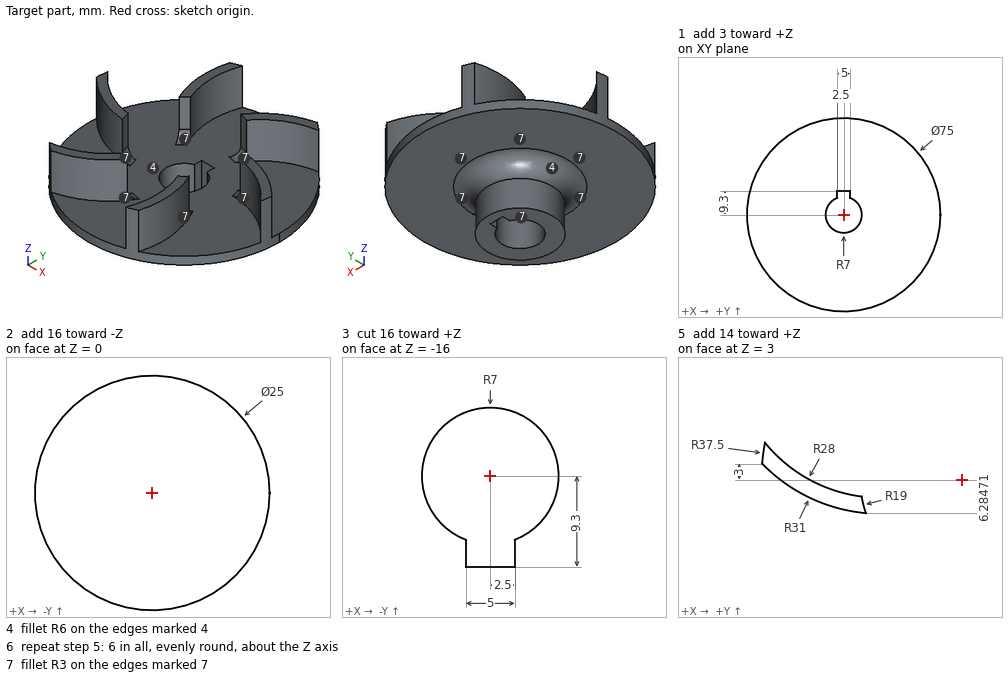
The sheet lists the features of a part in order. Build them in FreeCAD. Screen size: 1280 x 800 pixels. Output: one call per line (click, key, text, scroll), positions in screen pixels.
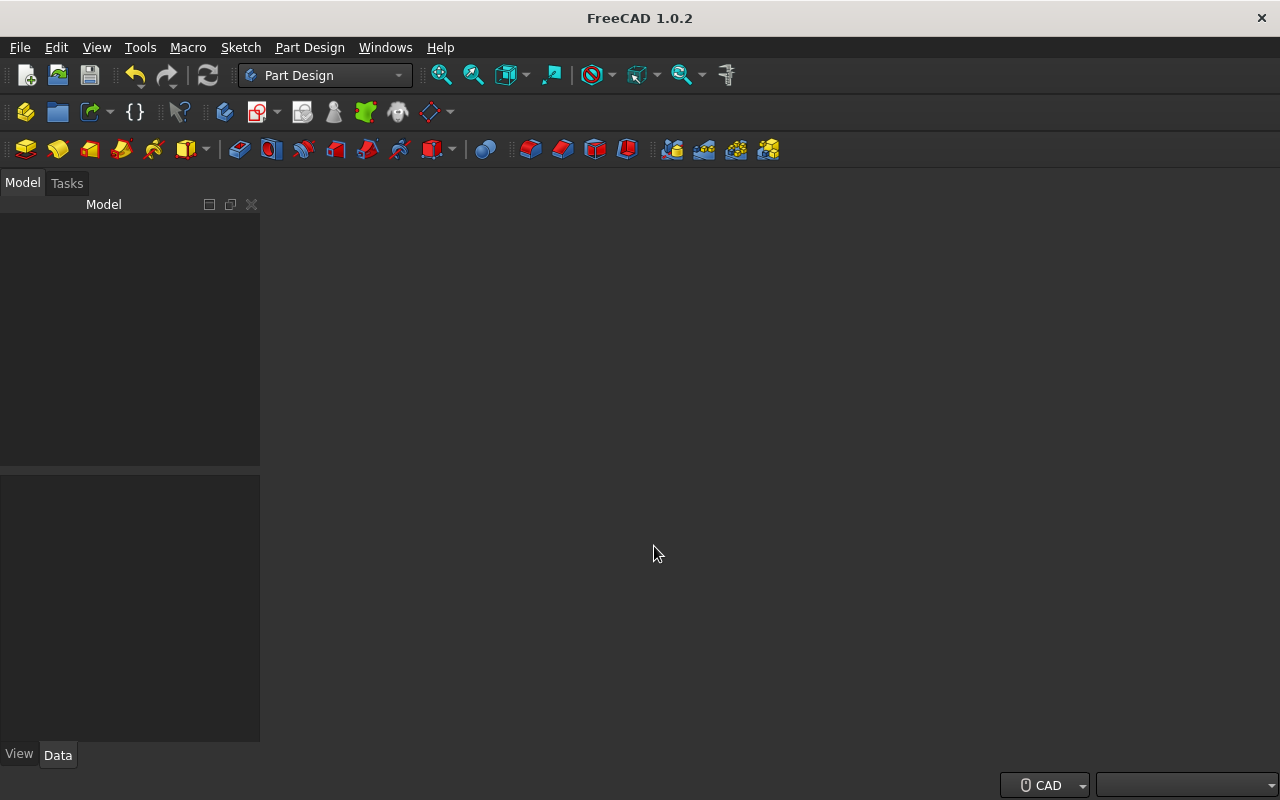
key(ctrl+n)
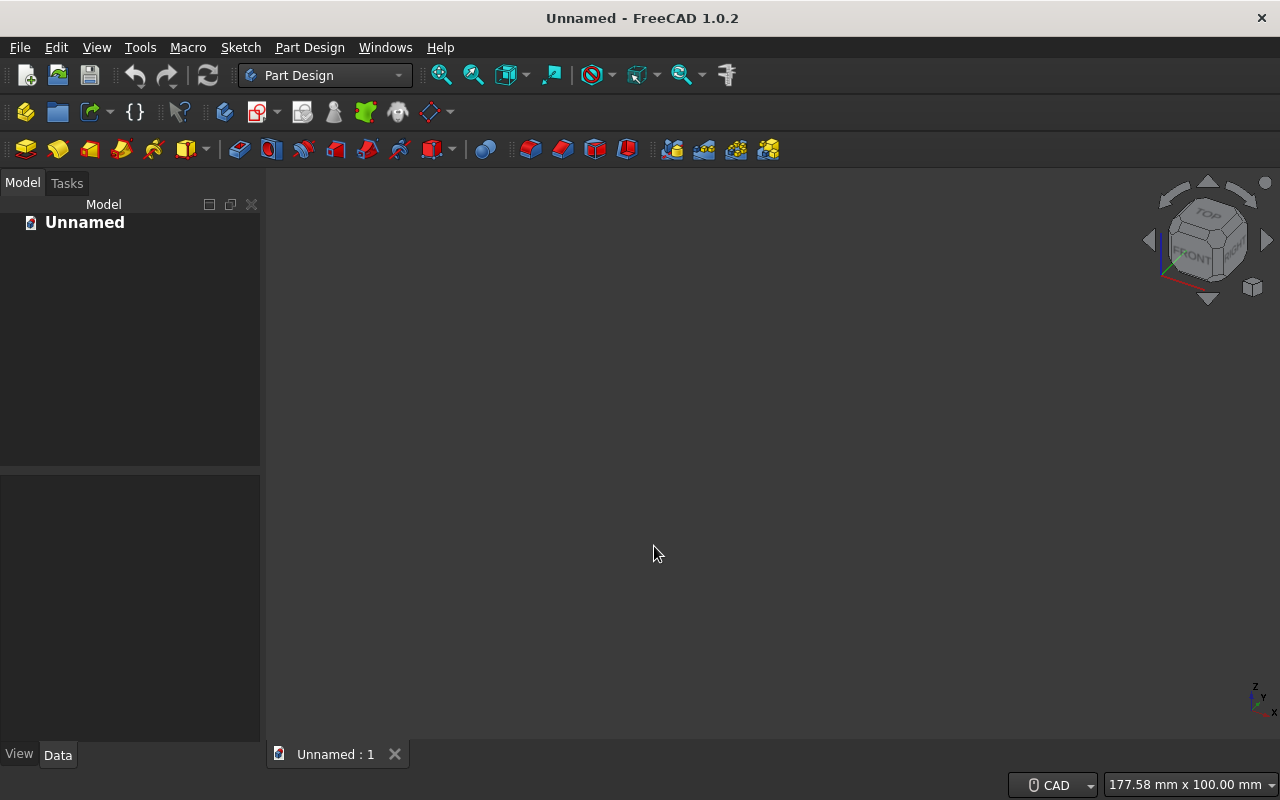
click(258, 112)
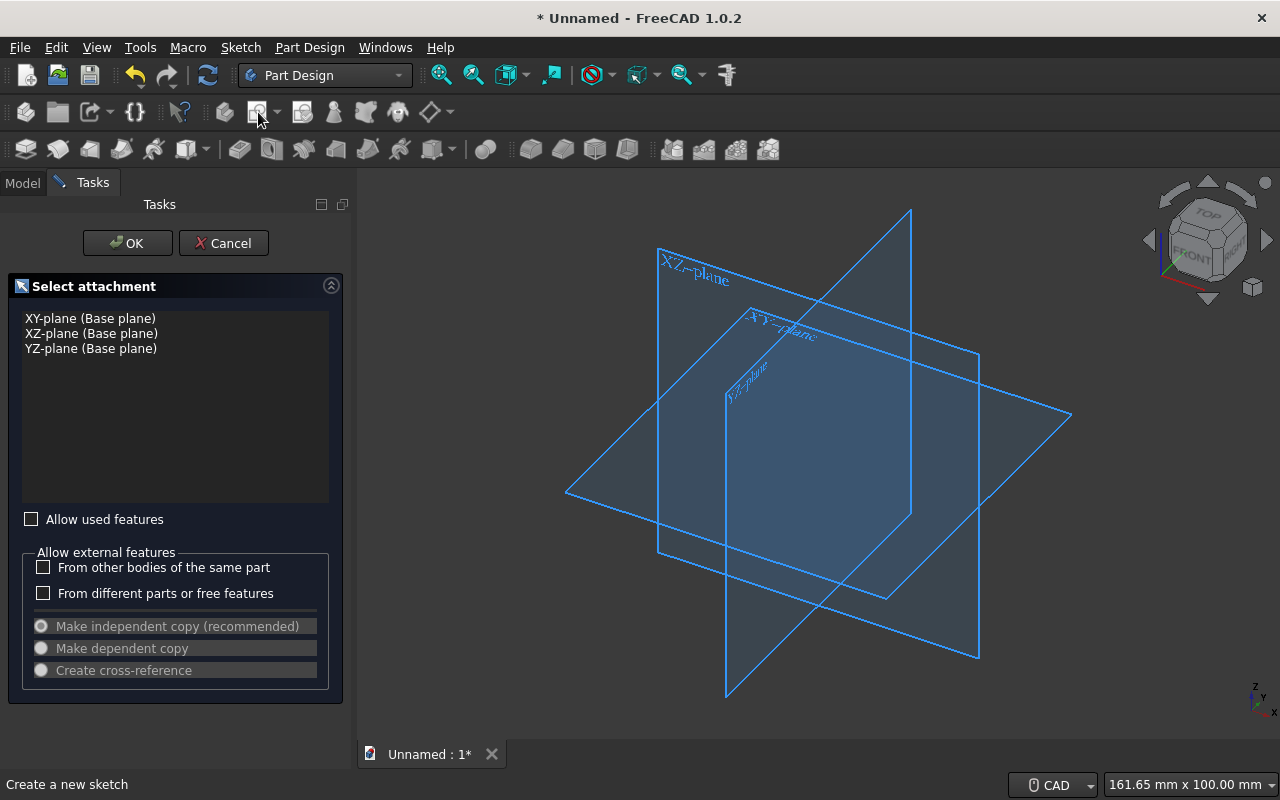
click(82, 318)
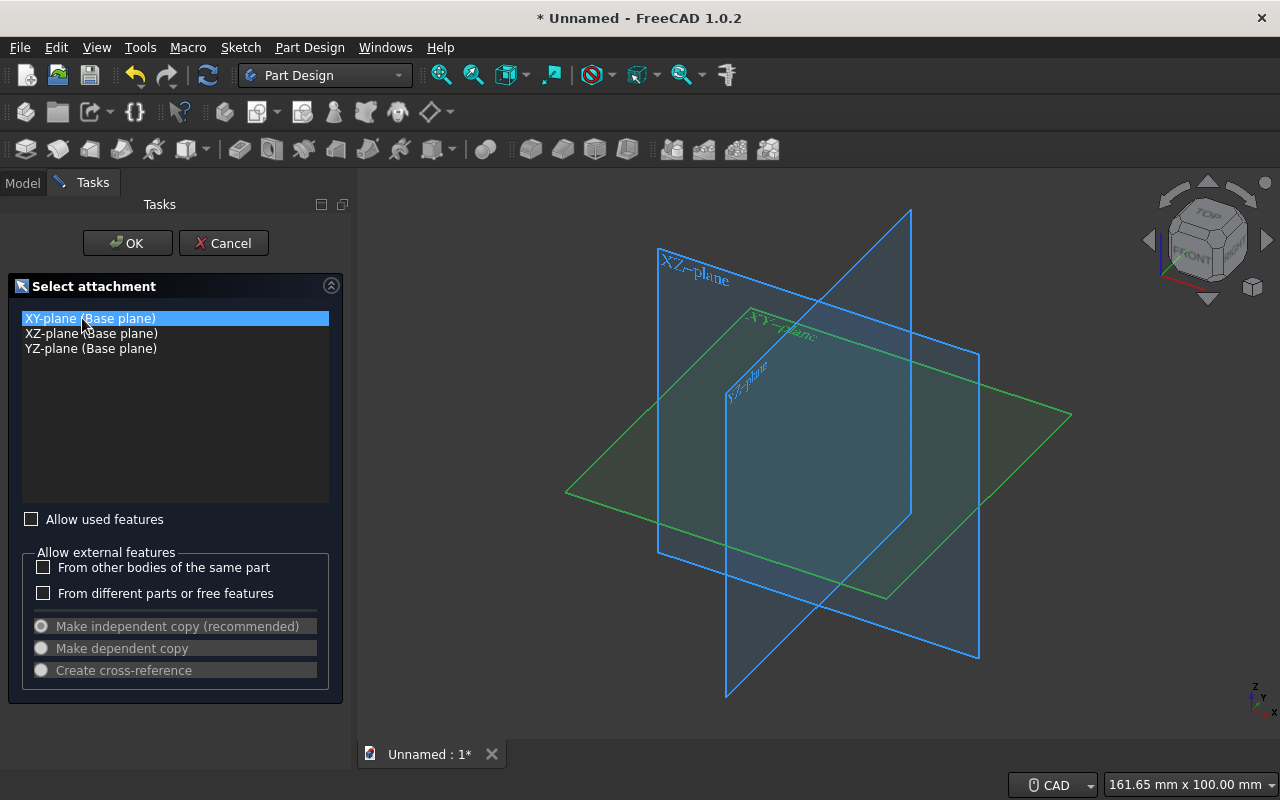
click(128, 243)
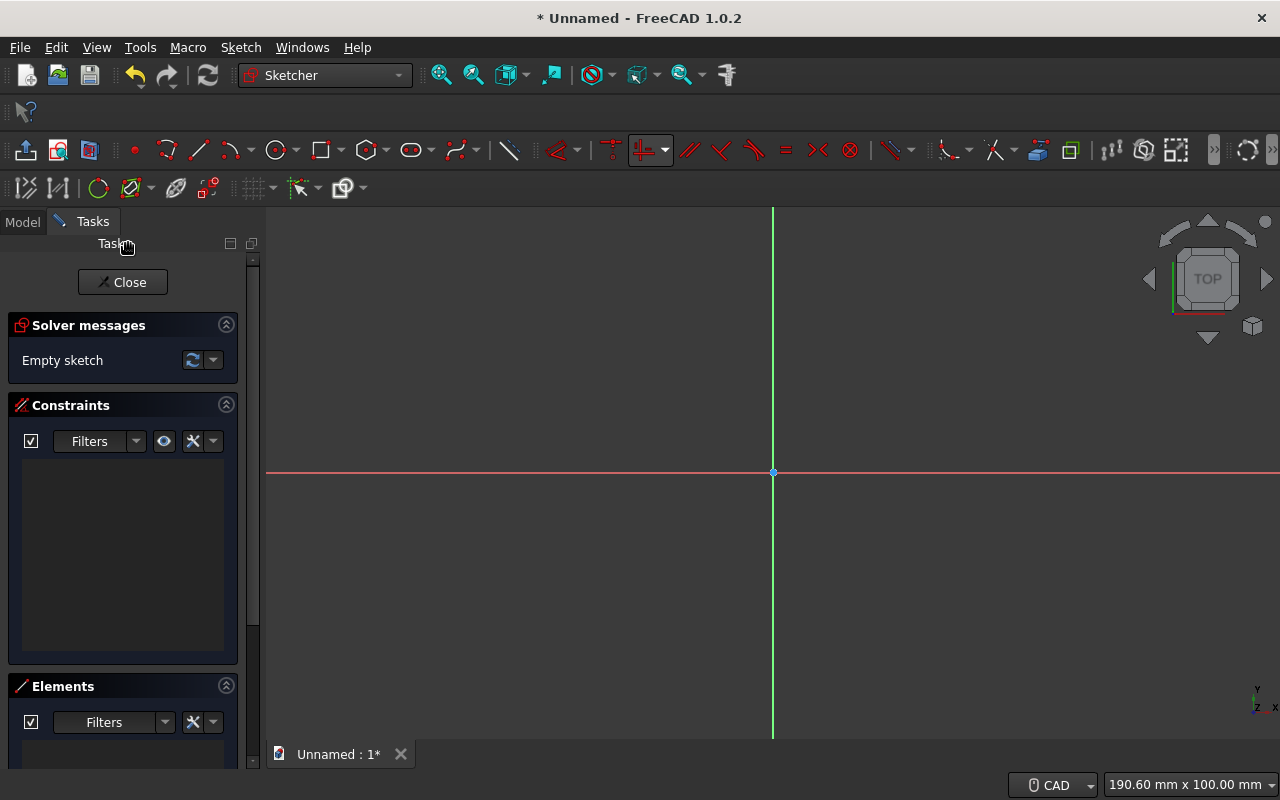
key(g)
key(m)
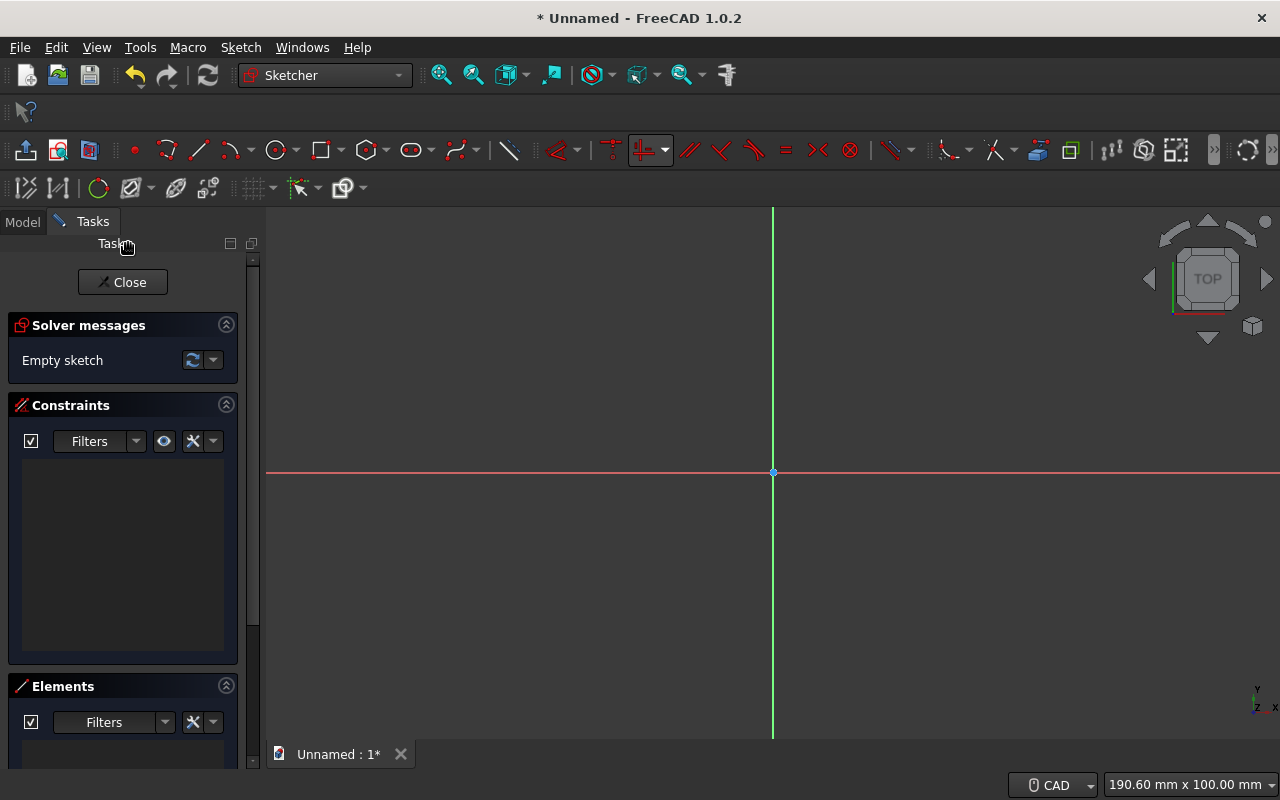
click(760, 438)
click(760, 424)
click(786, 424)
click(786, 438)
right_click(786, 438)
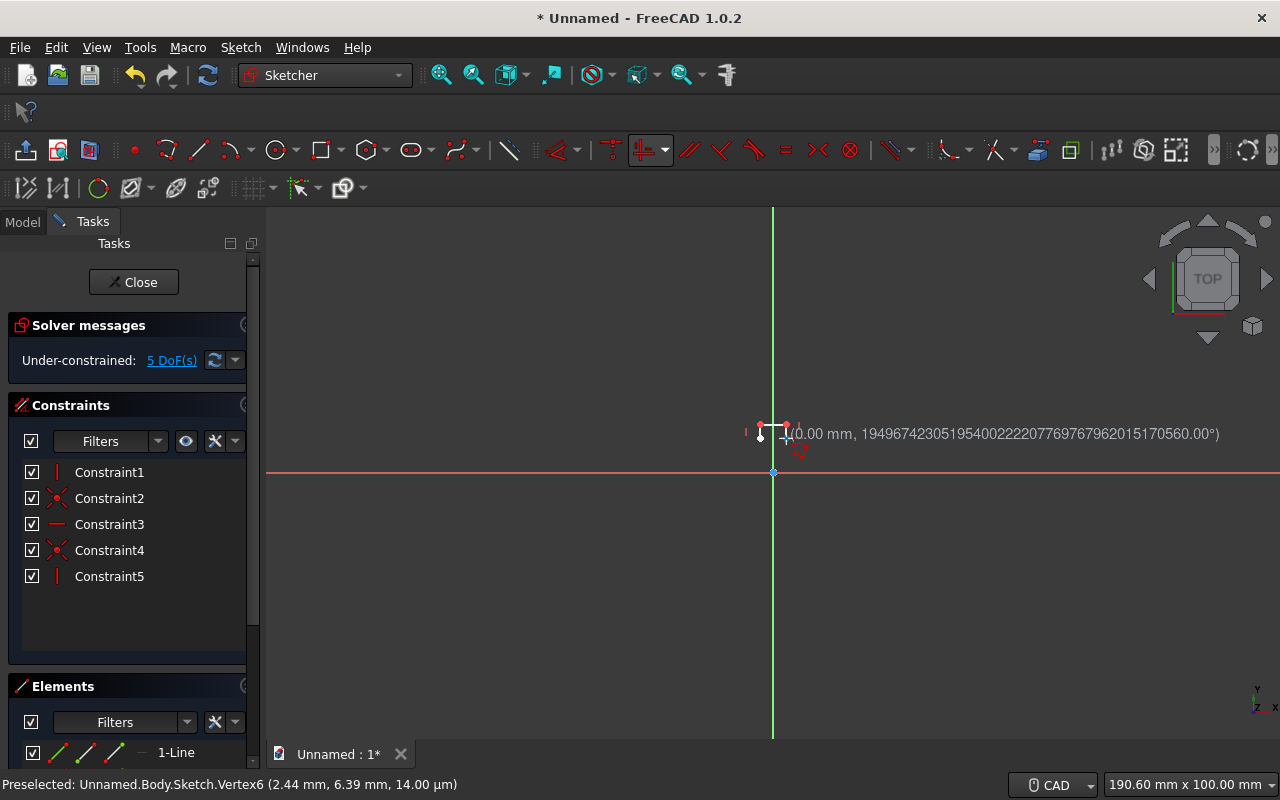
key(g)
key(3)
key(a)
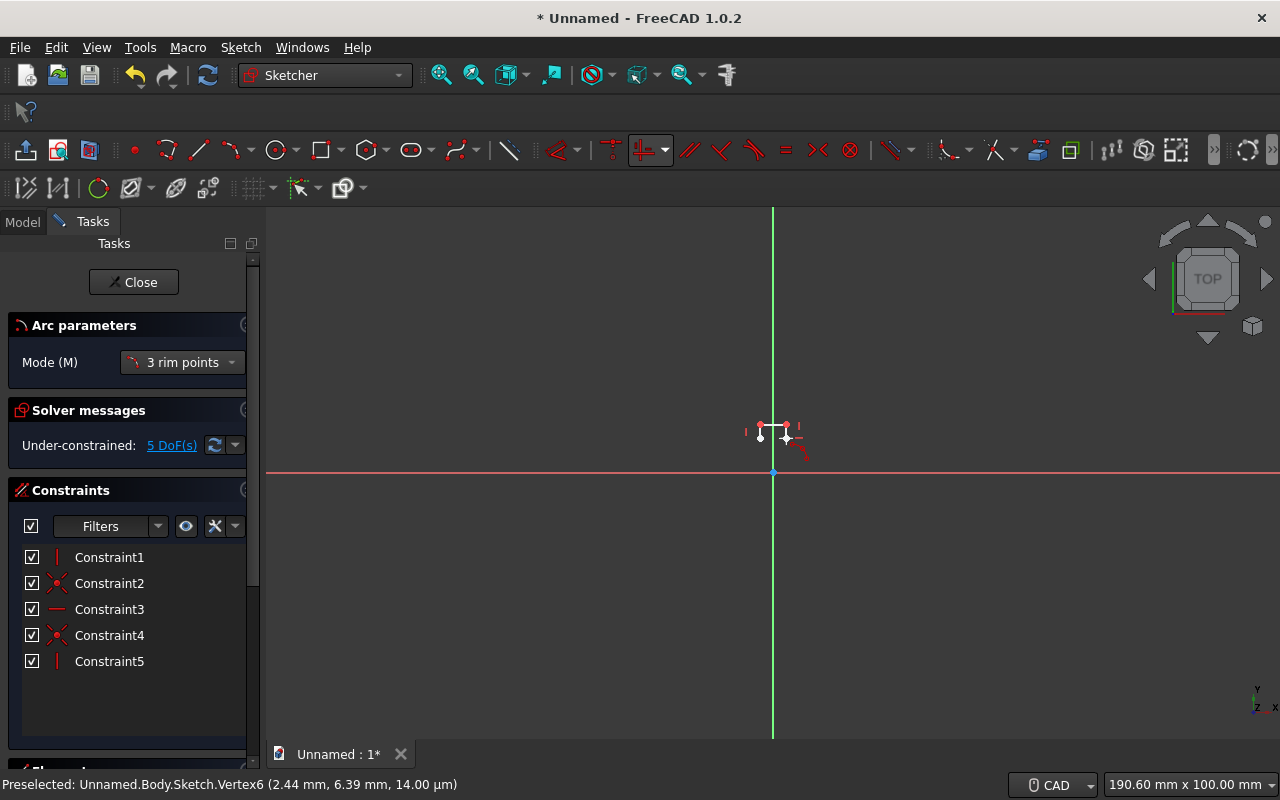
scroll(786, 438, up, 4)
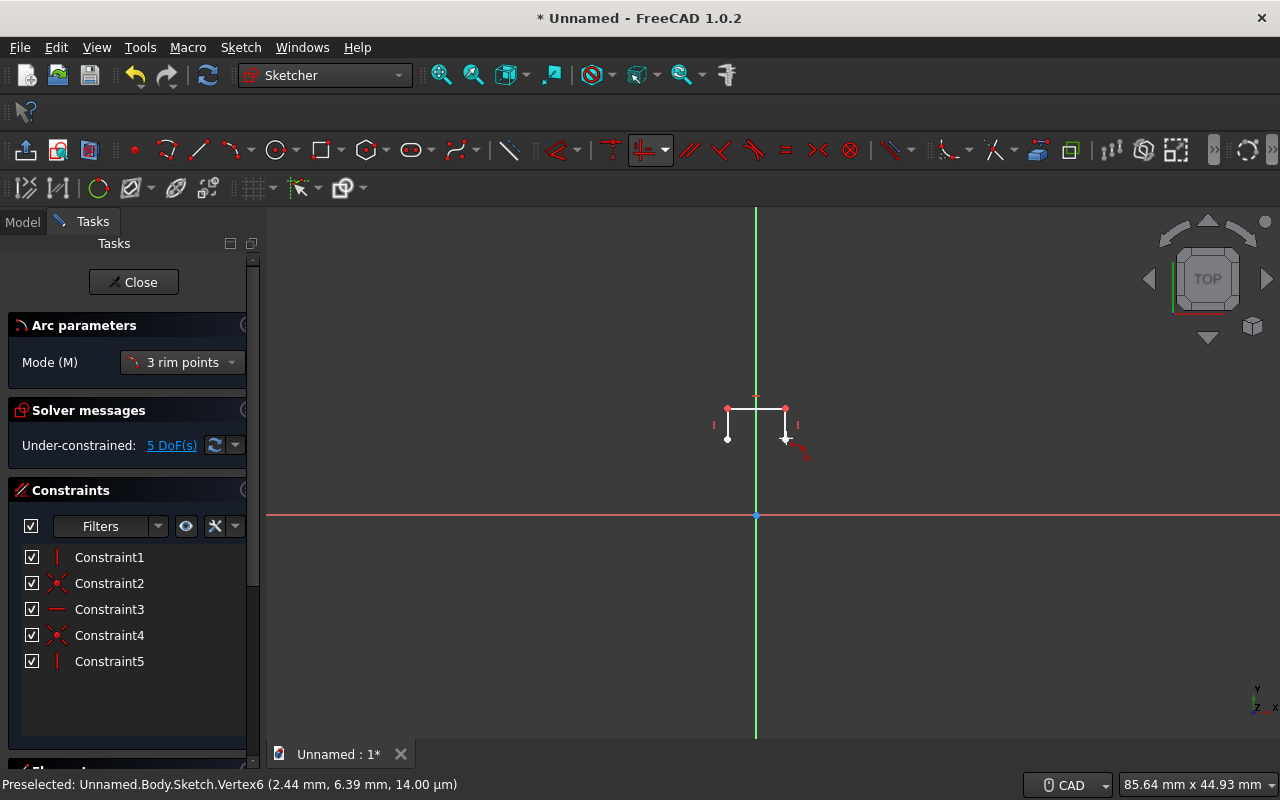
click(785, 440)
click(728, 440)
click(713, 586)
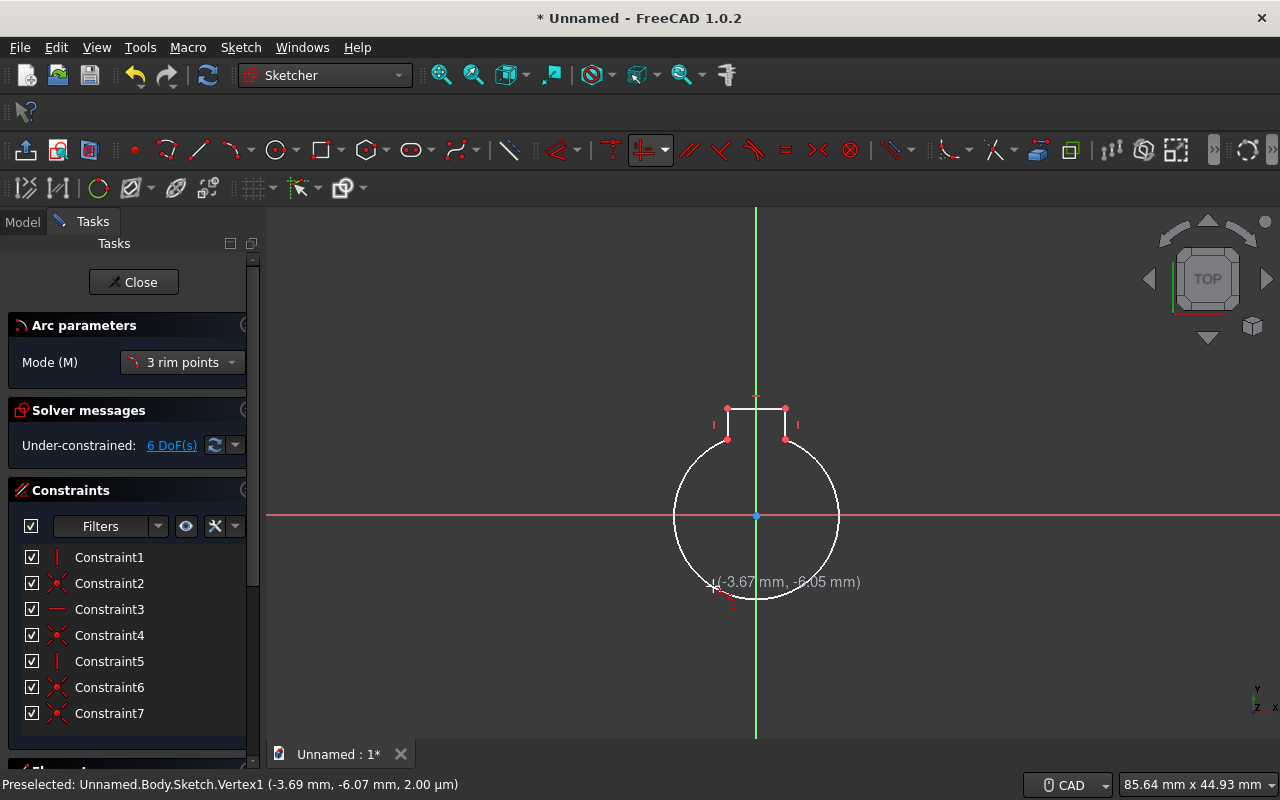
key(g)
key(c)